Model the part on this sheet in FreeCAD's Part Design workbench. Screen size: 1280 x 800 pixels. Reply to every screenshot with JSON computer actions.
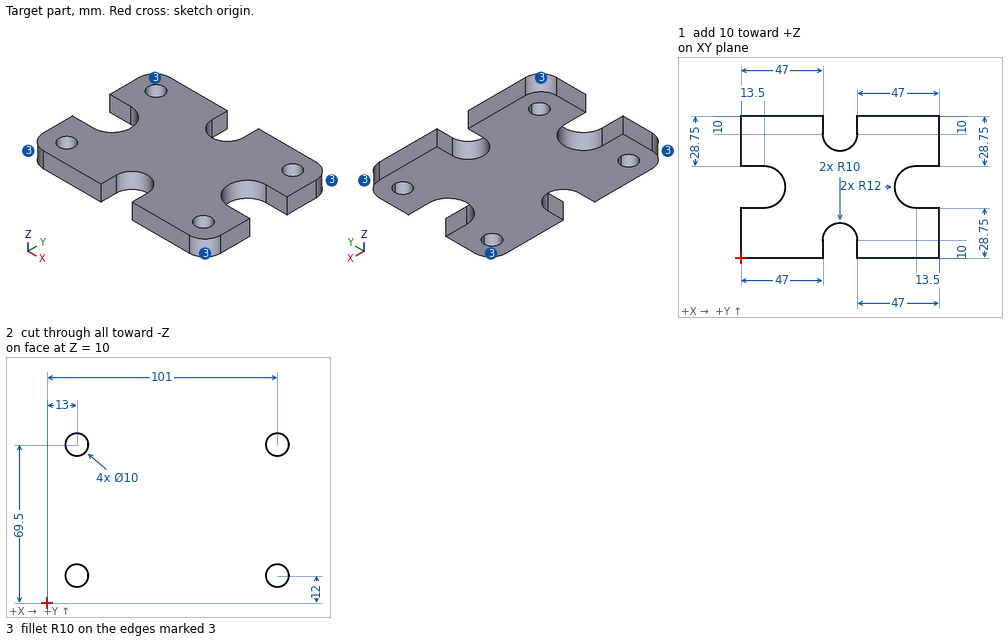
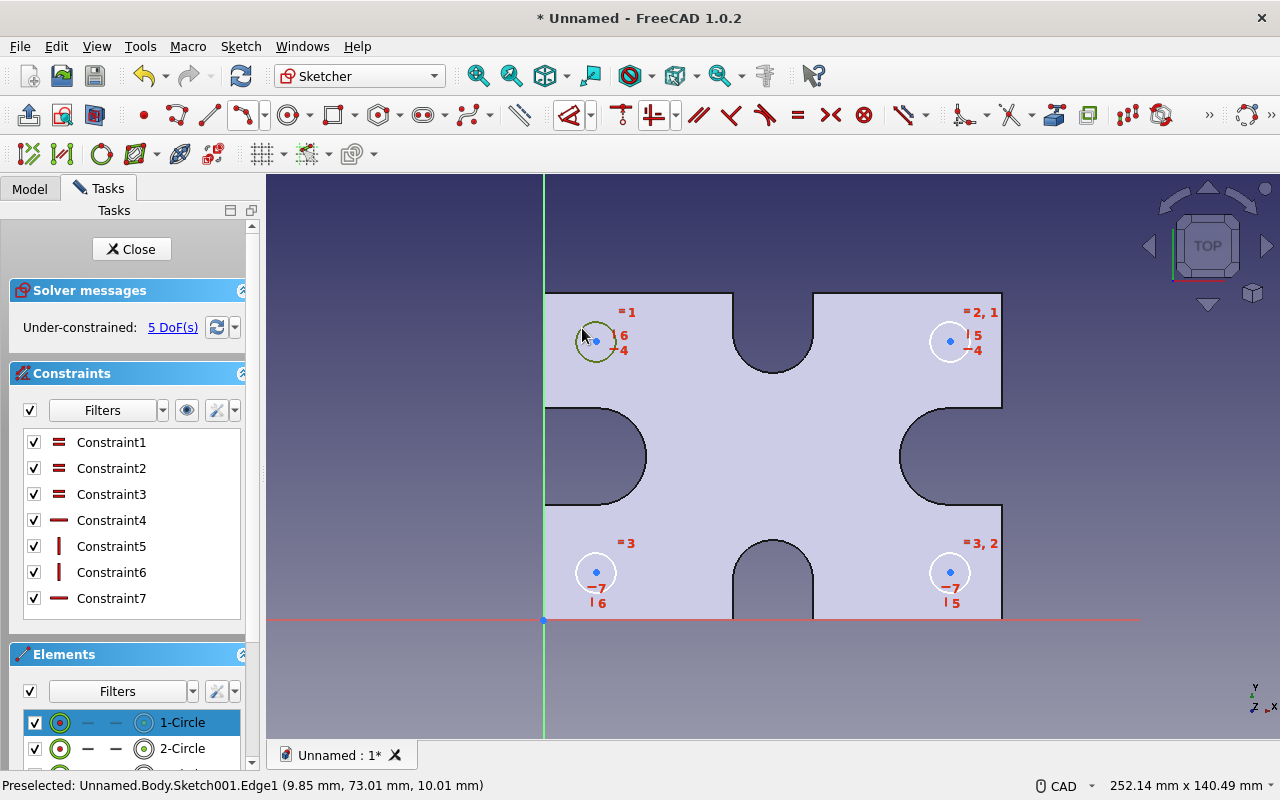
{"action": "key", "text": "k o"}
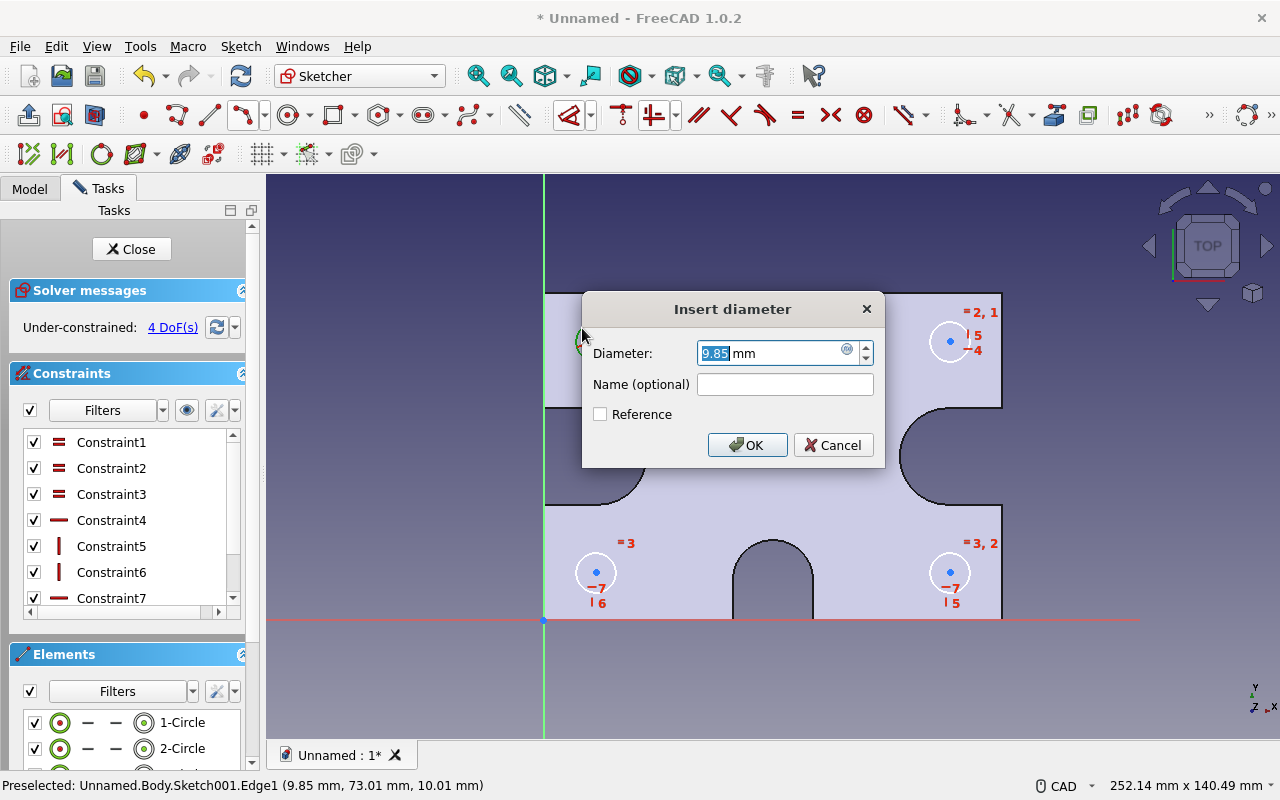
{"action": "type", "text": "10"}
{"action": "key", "text": "Return"}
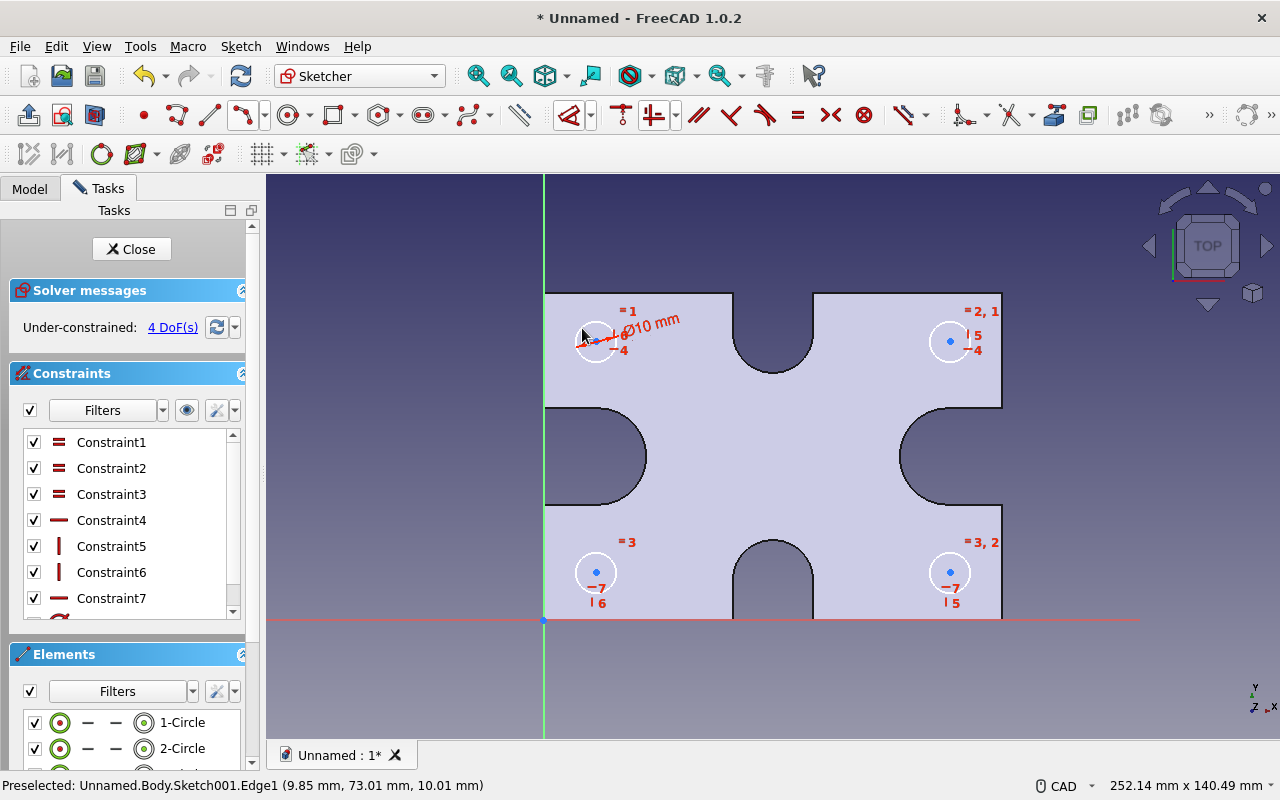
{"action": "left_click", "coordinate": [596, 342]}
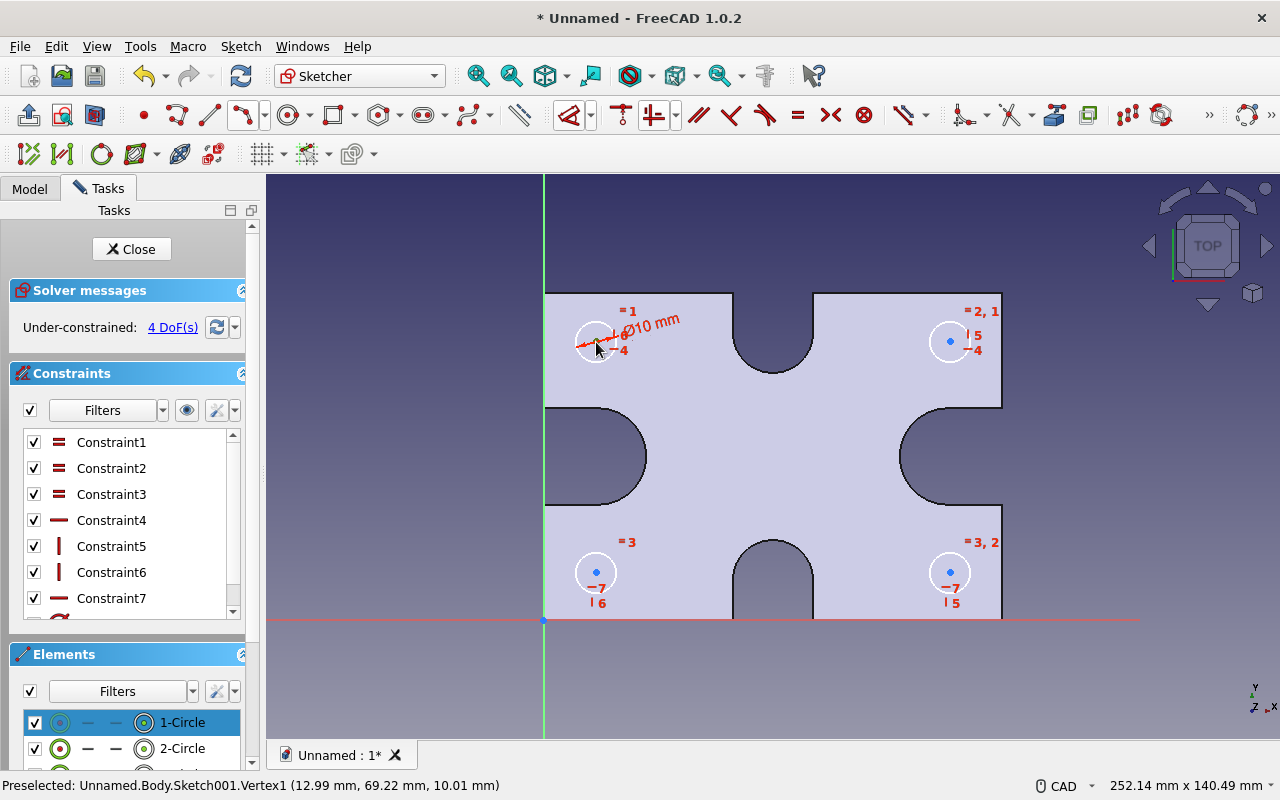
{"action": "key", "text": "l"}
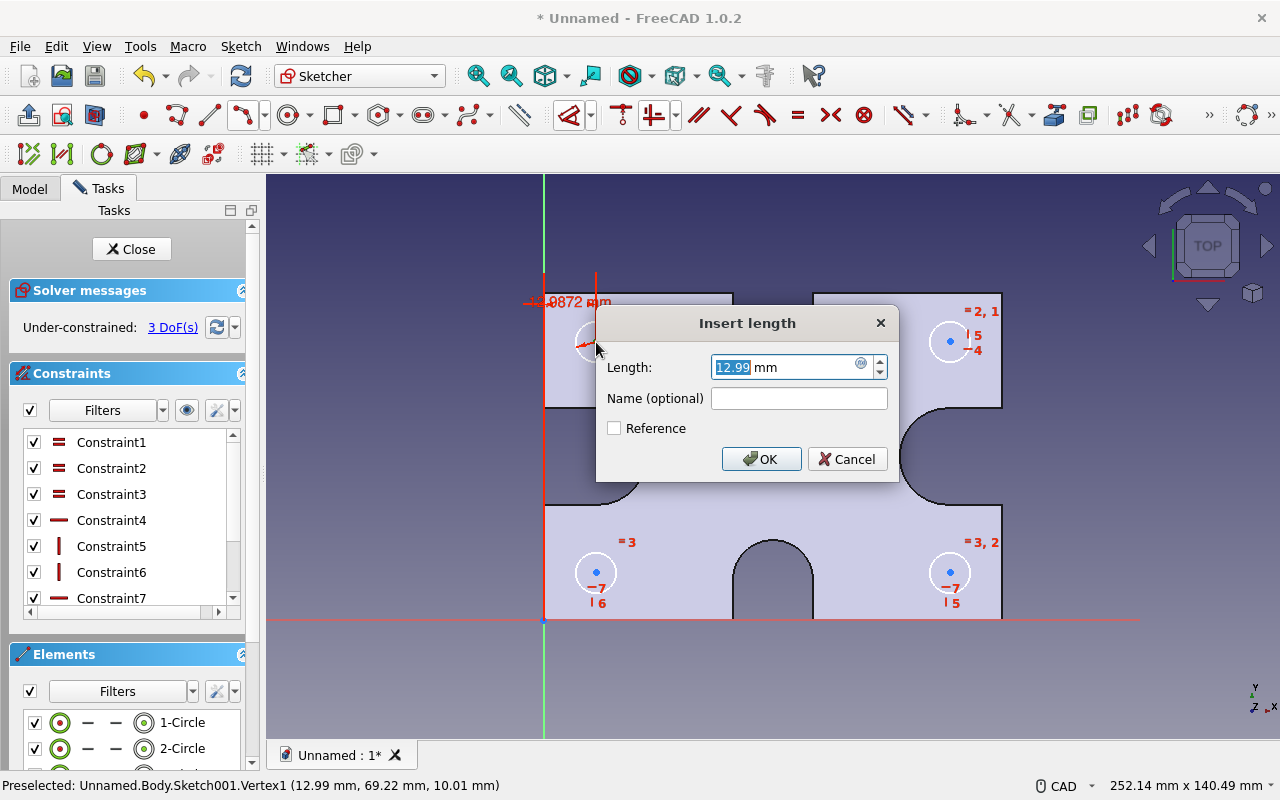
{"action": "type", "text": "13"}
{"action": "key", "text": "Return"}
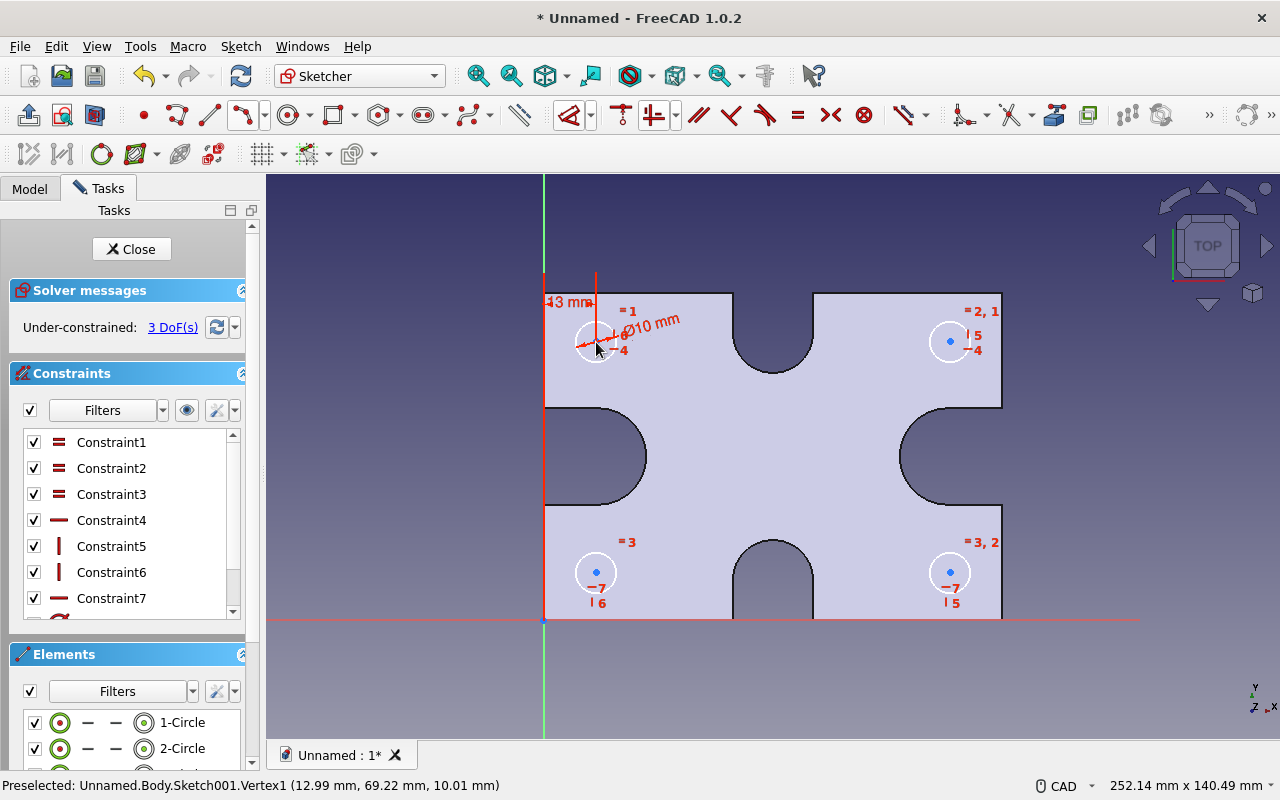
{"action": "left_click", "coordinate": [950, 573]}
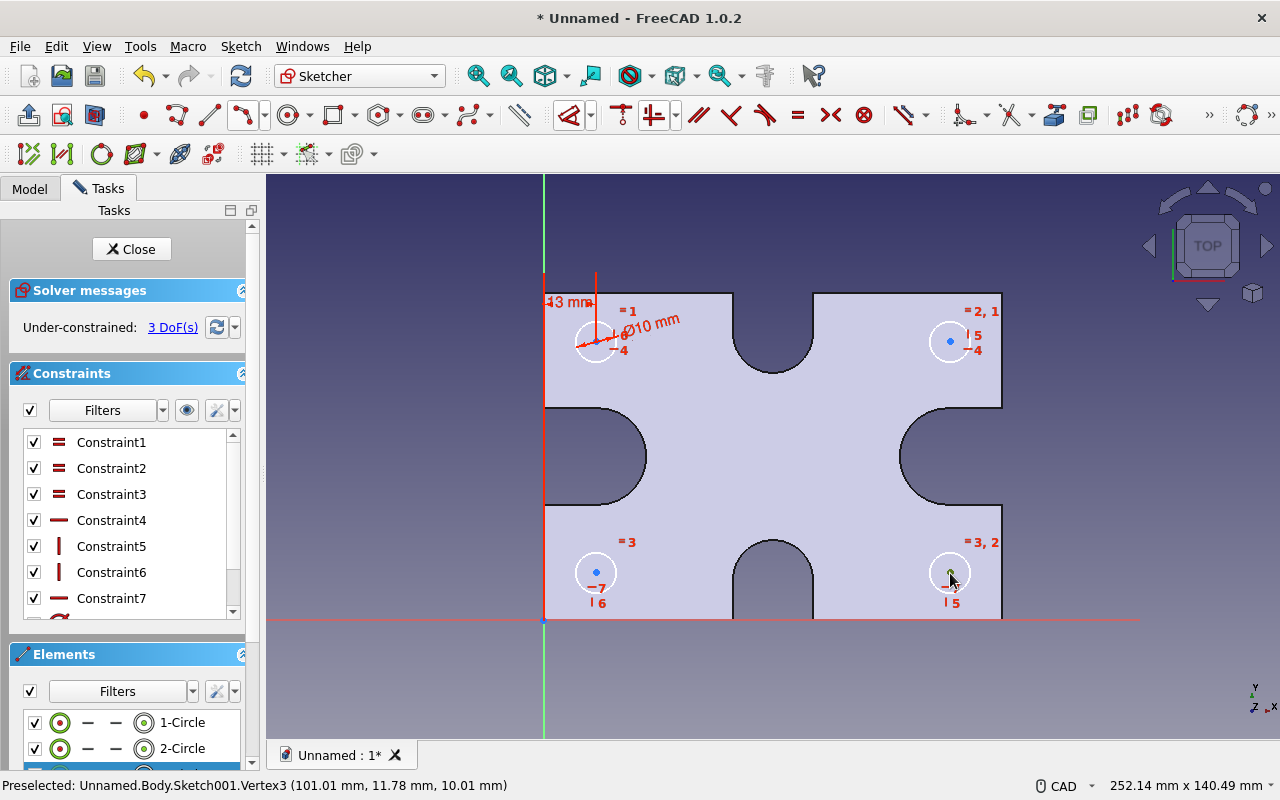
{"action": "key", "text": "i"}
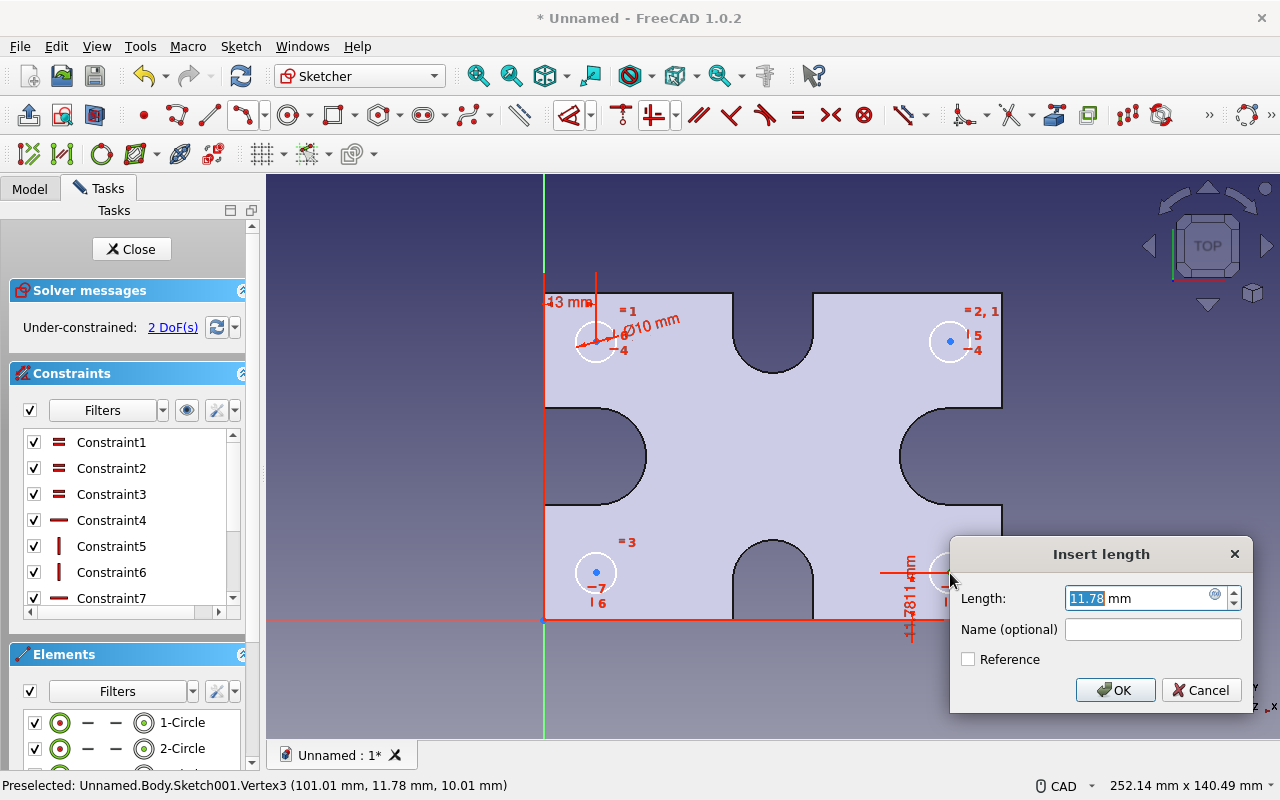
{"action": "type", "text": "12"}
{"action": "key", "text": "Return"}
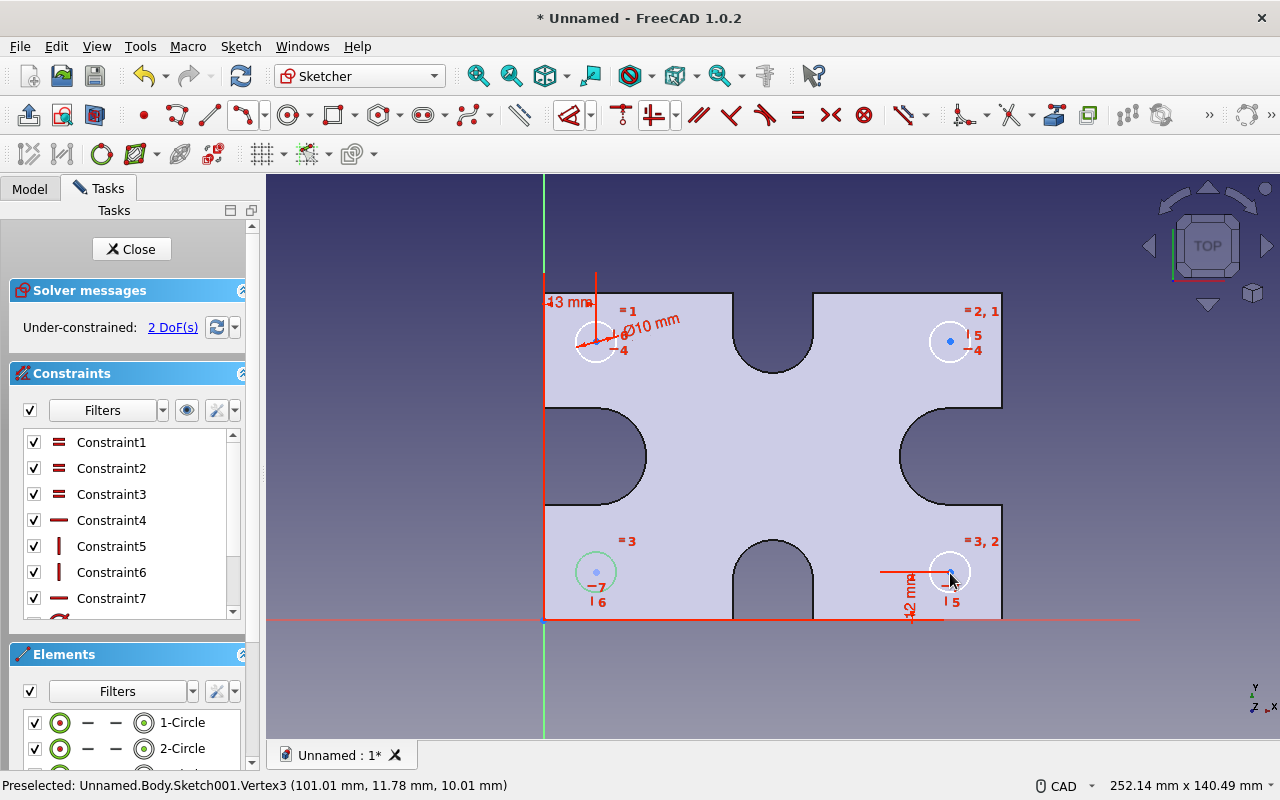
{"action": "left_click", "coordinate": [950, 342]}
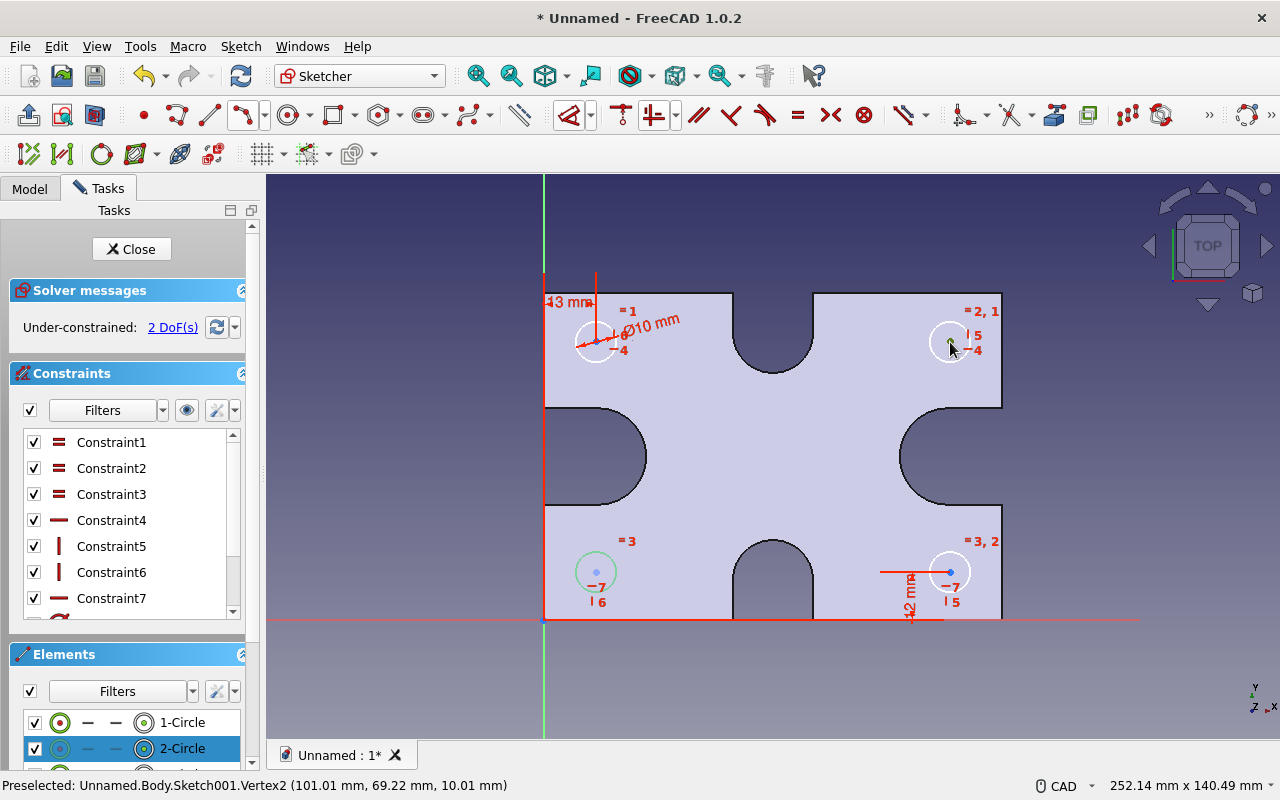
{"action": "key", "text": "l"}